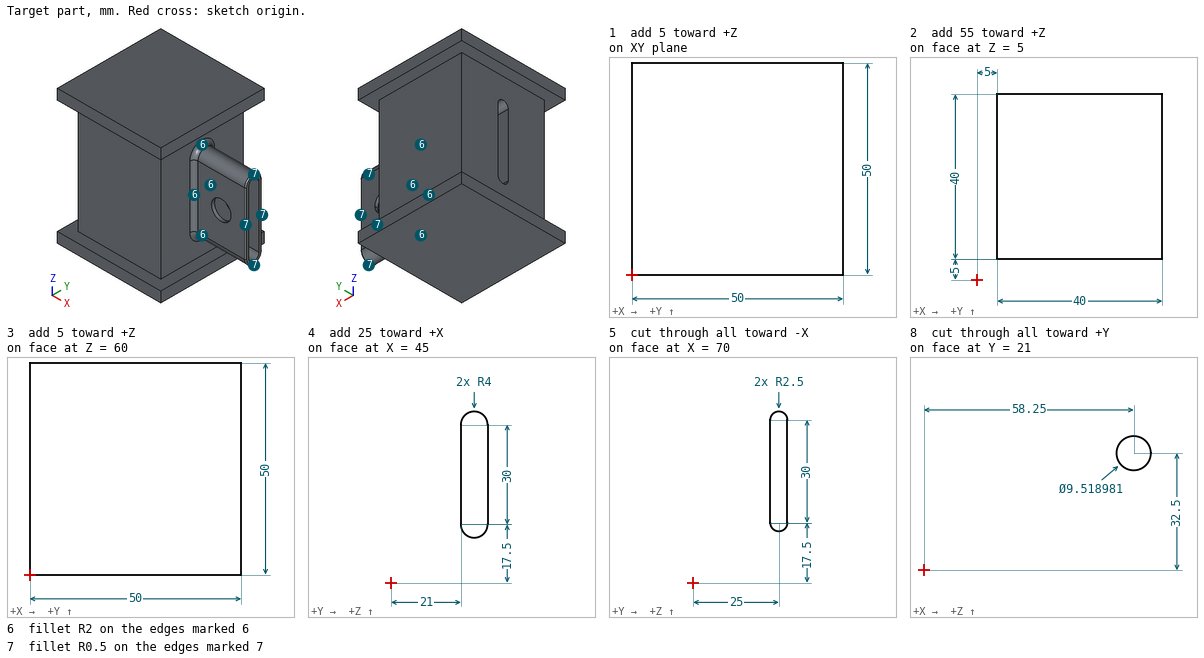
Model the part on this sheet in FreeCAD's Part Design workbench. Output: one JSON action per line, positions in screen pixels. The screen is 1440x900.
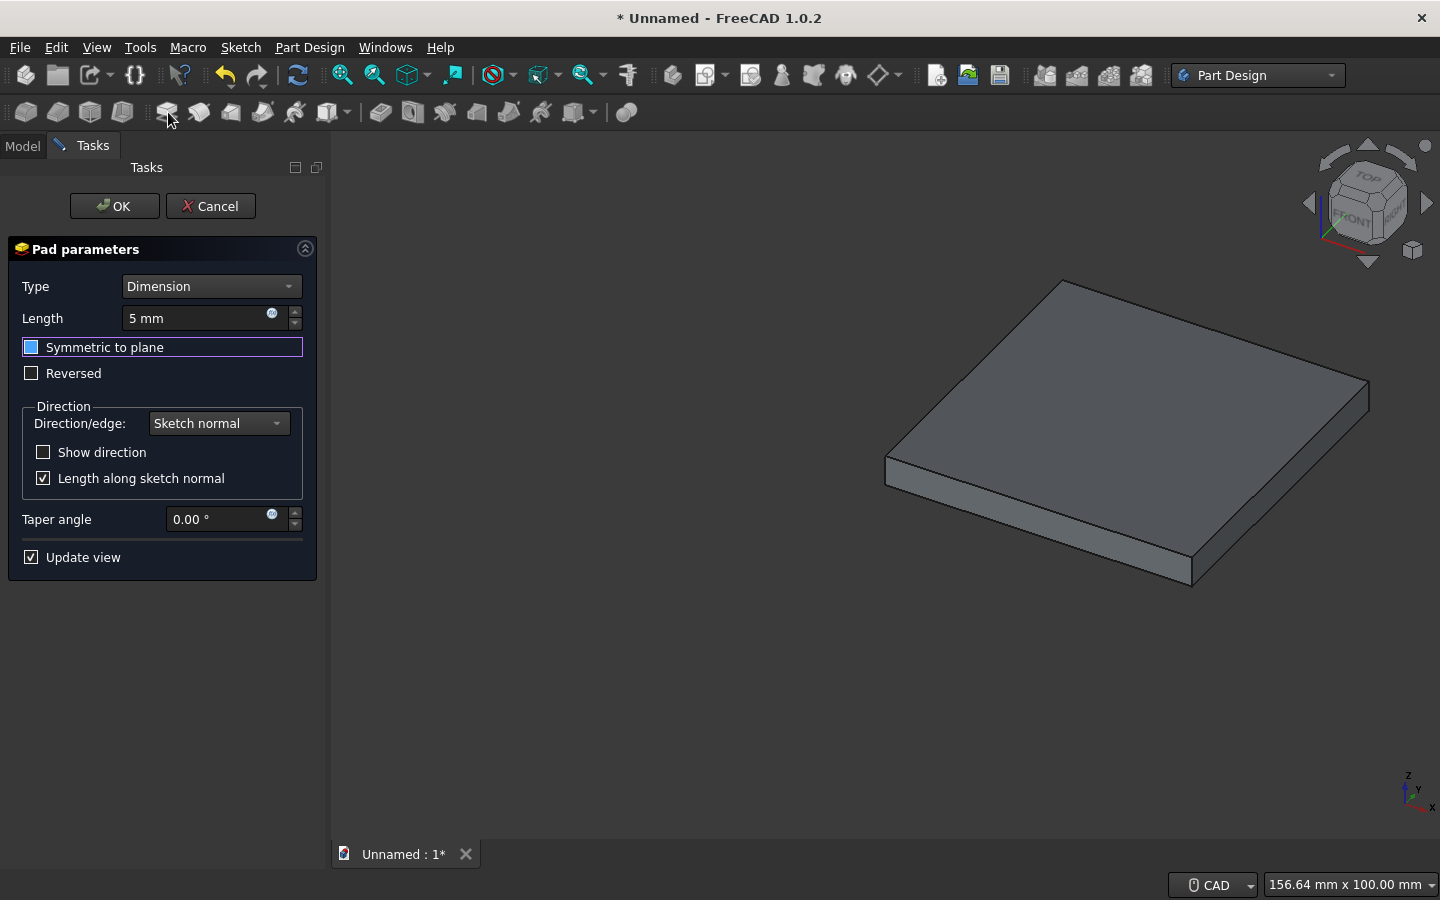
{"action": "left_click", "coordinate": [115, 206]}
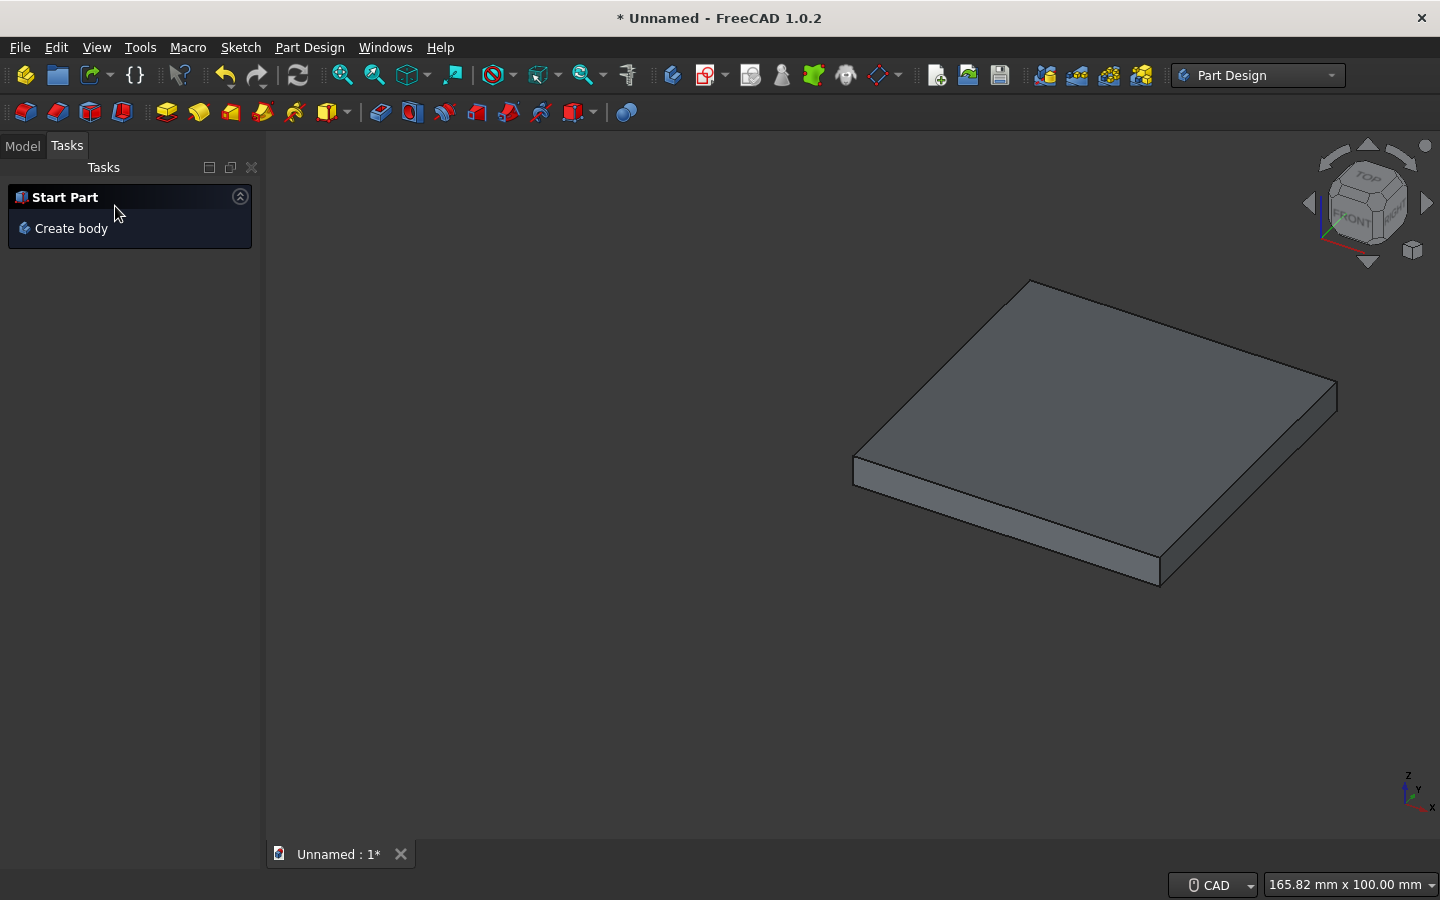
{"action": "left_click", "coordinate": [344, 76]}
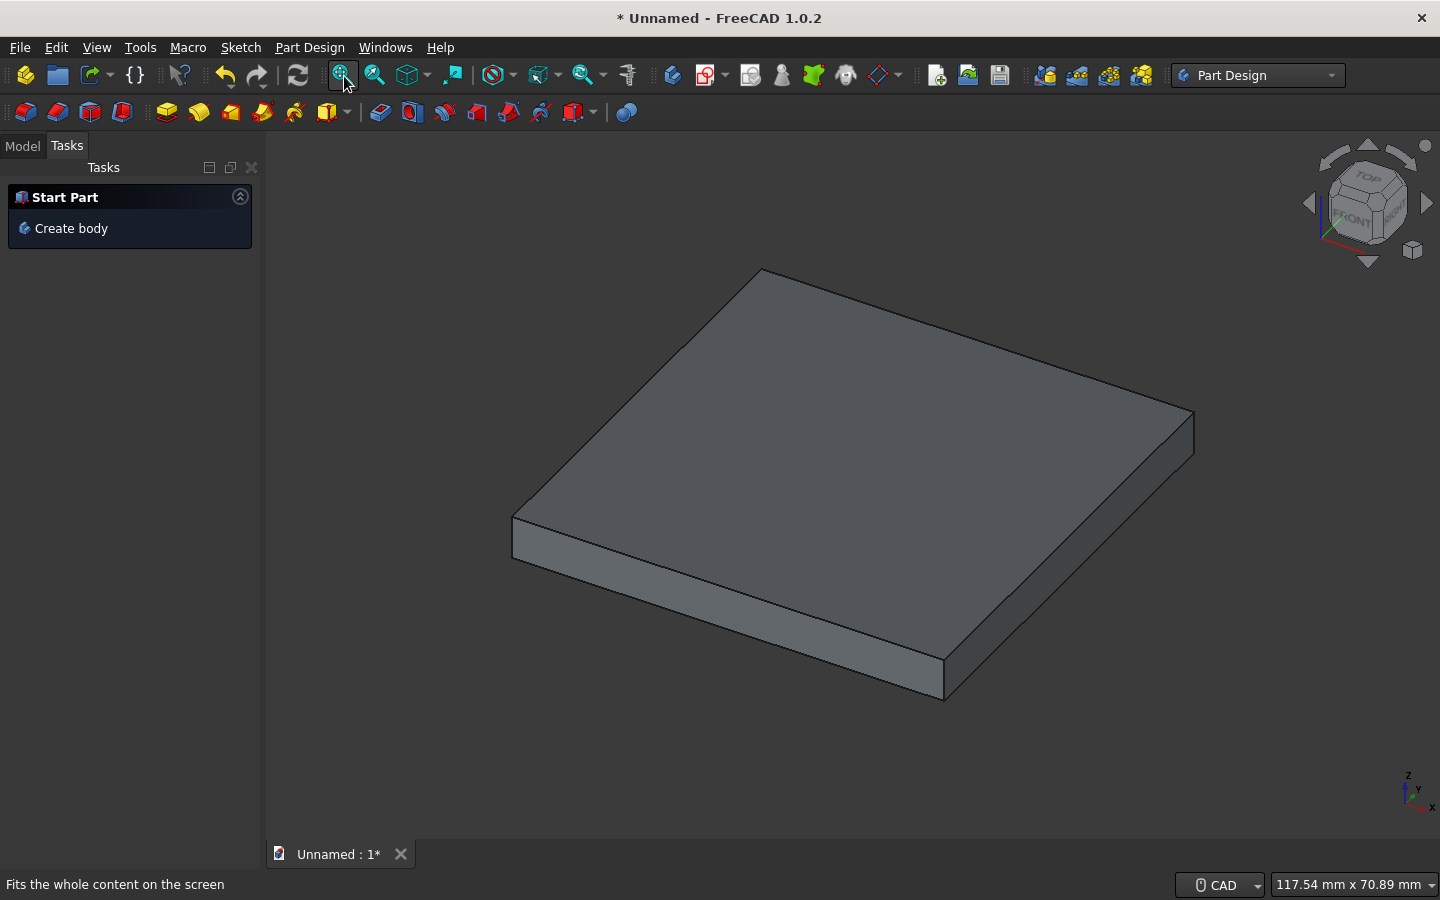
{"action": "left_click", "coordinate": [853, 464]}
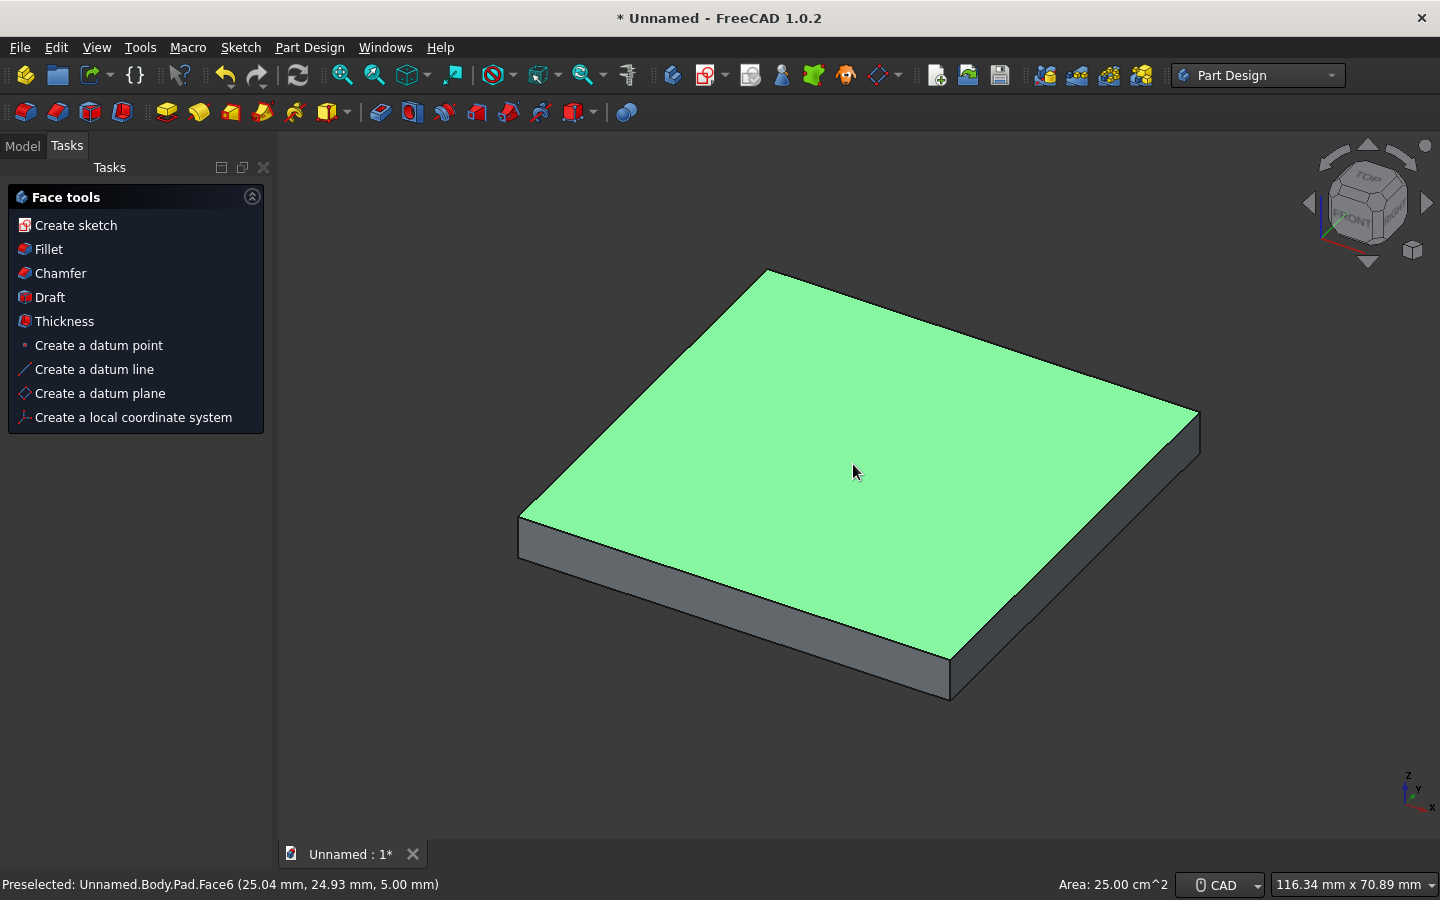
{"action": "left_click", "coordinate": [706, 76]}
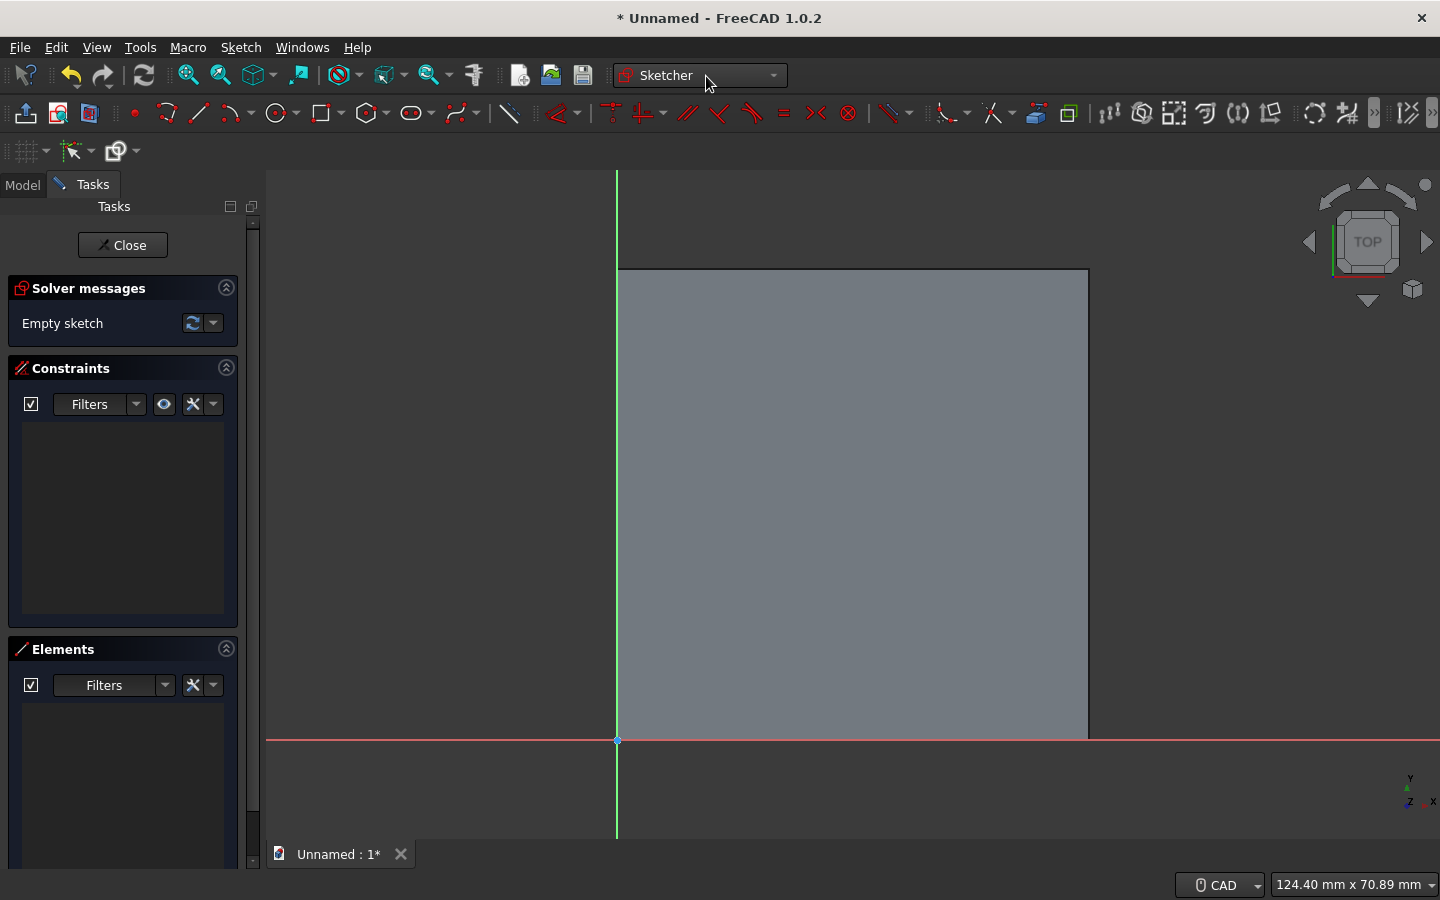
{"action": "left_click", "coordinate": [322, 114]}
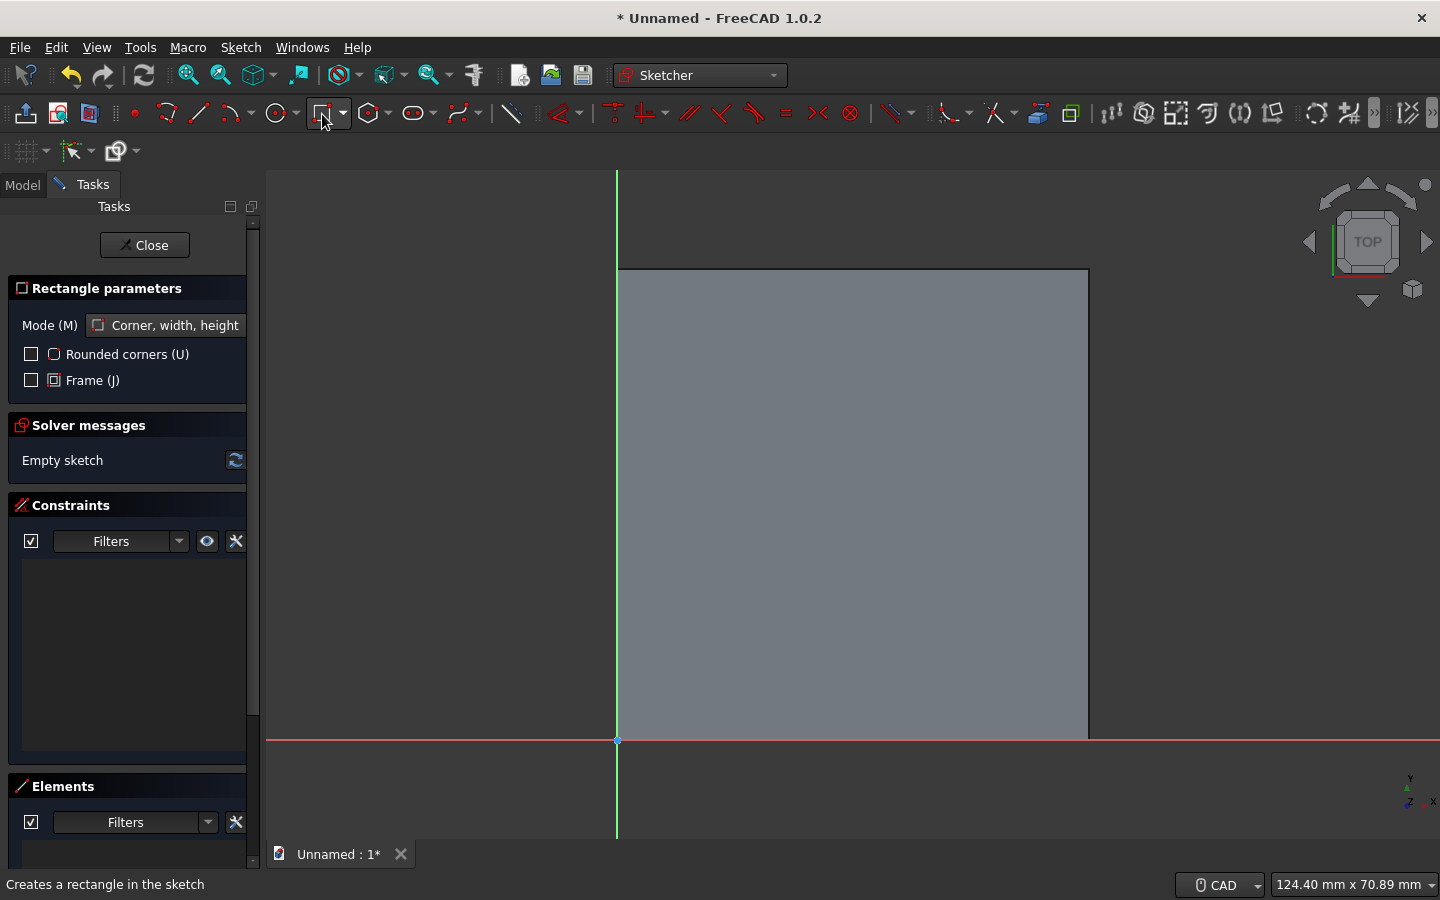
{"action": "left_click", "coordinate": [664, 316]}
{"action": "left_click", "coordinate": [1042, 693]}
{"action": "key", "text": "Escape"}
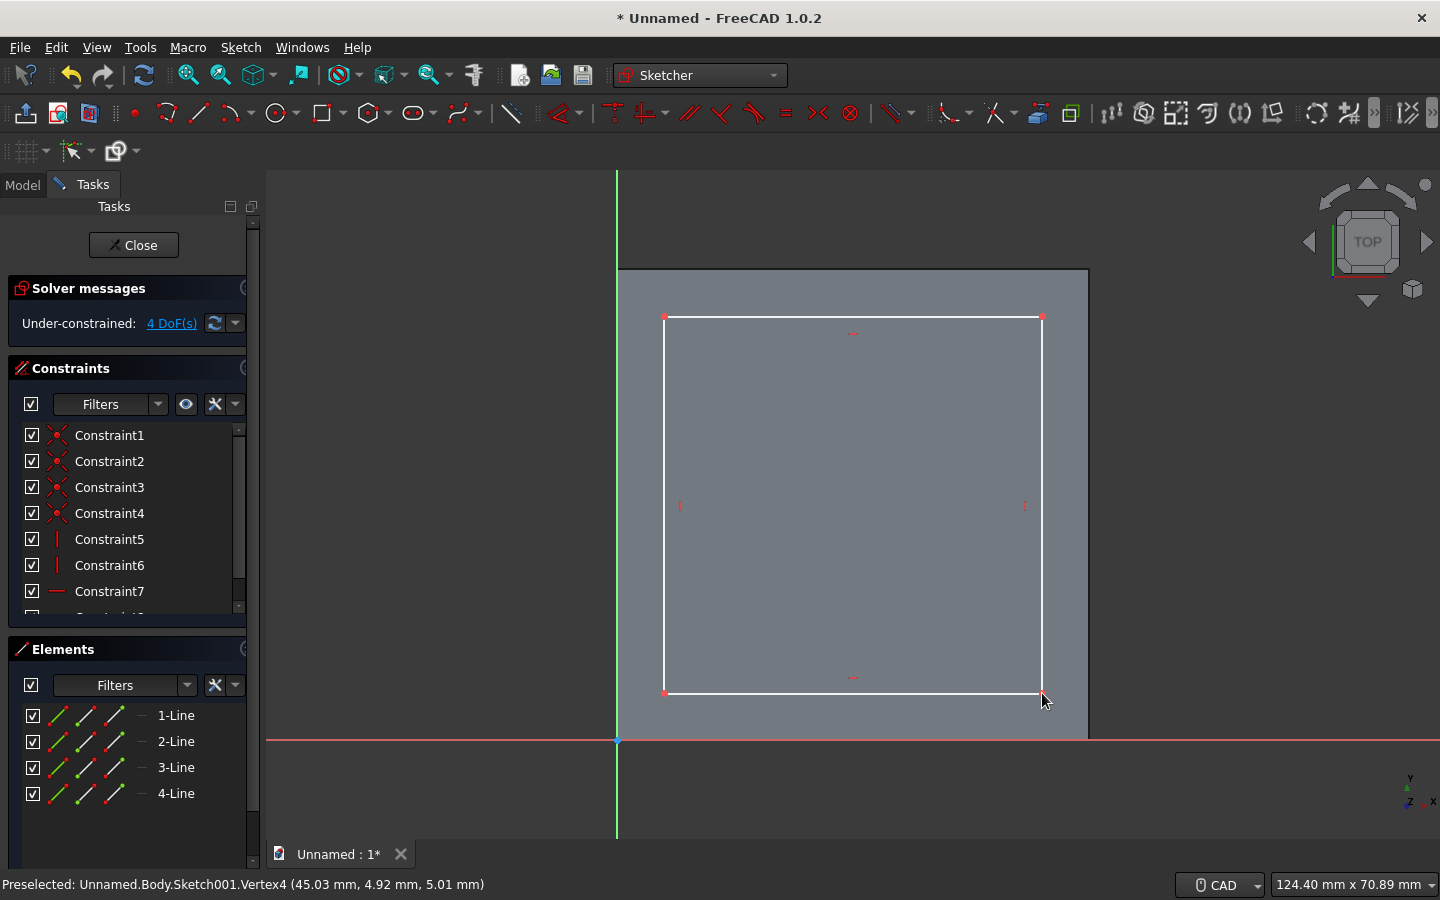
{"action": "left_click", "coordinate": [558, 114]}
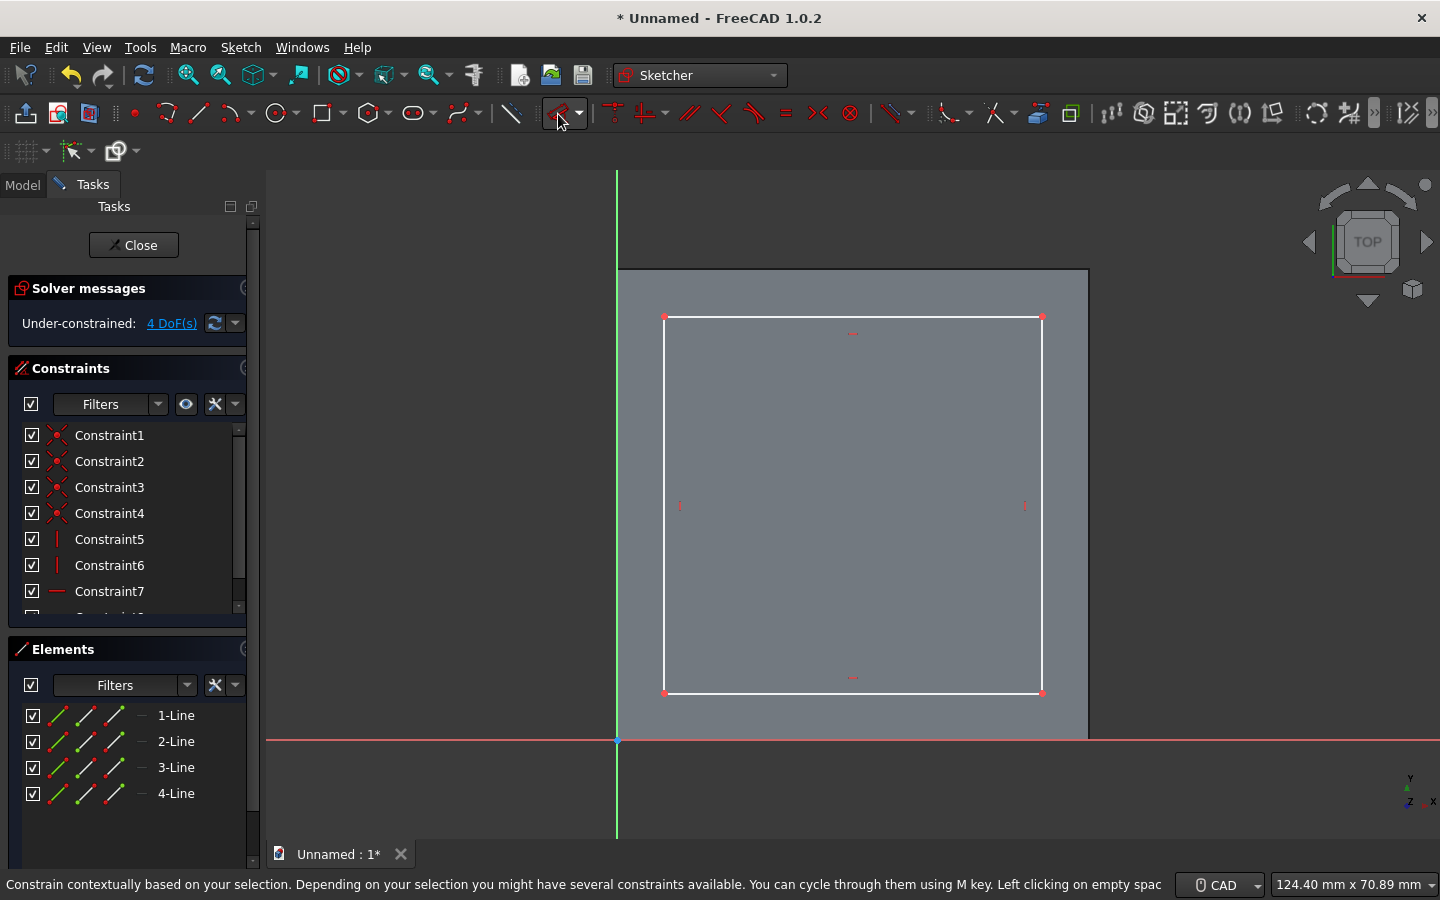
{"action": "left_click", "coordinate": [664, 430]}
{"action": "left_click", "coordinate": [698, 506]}